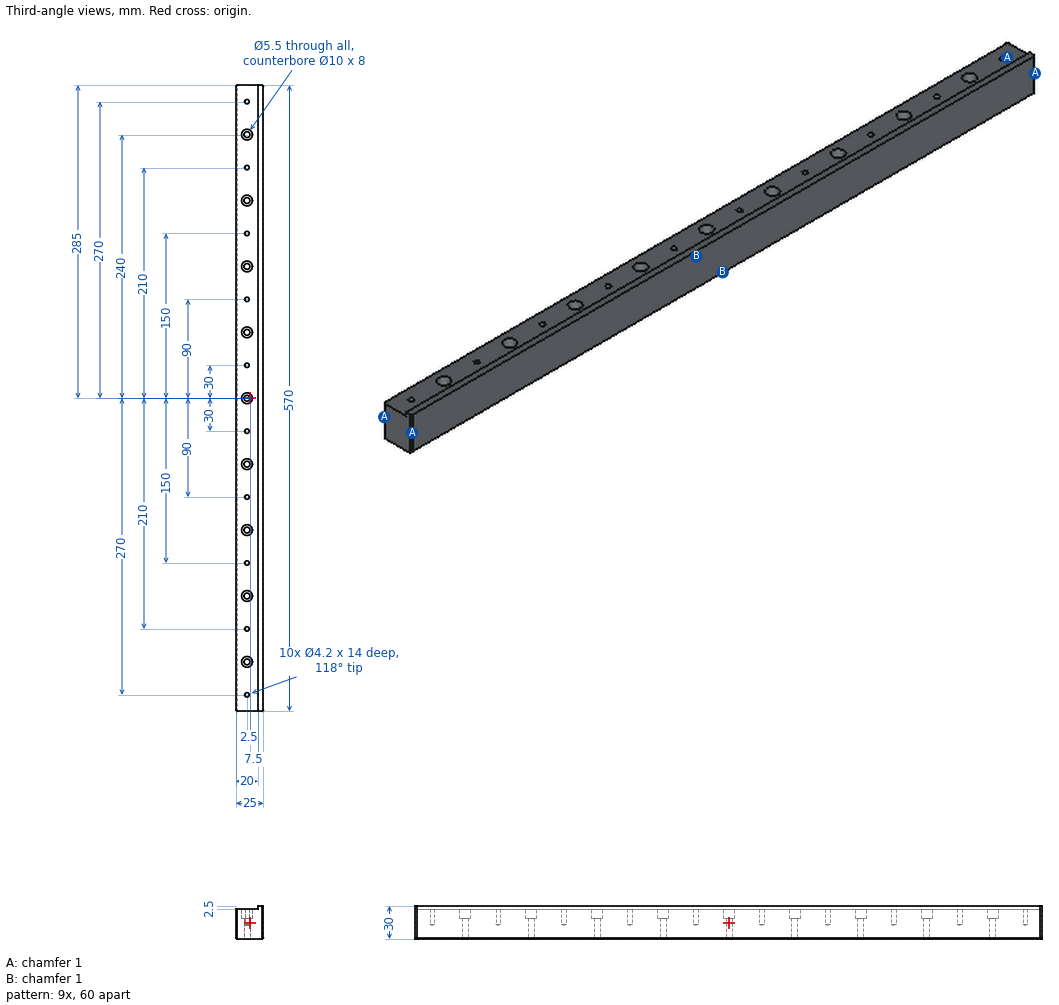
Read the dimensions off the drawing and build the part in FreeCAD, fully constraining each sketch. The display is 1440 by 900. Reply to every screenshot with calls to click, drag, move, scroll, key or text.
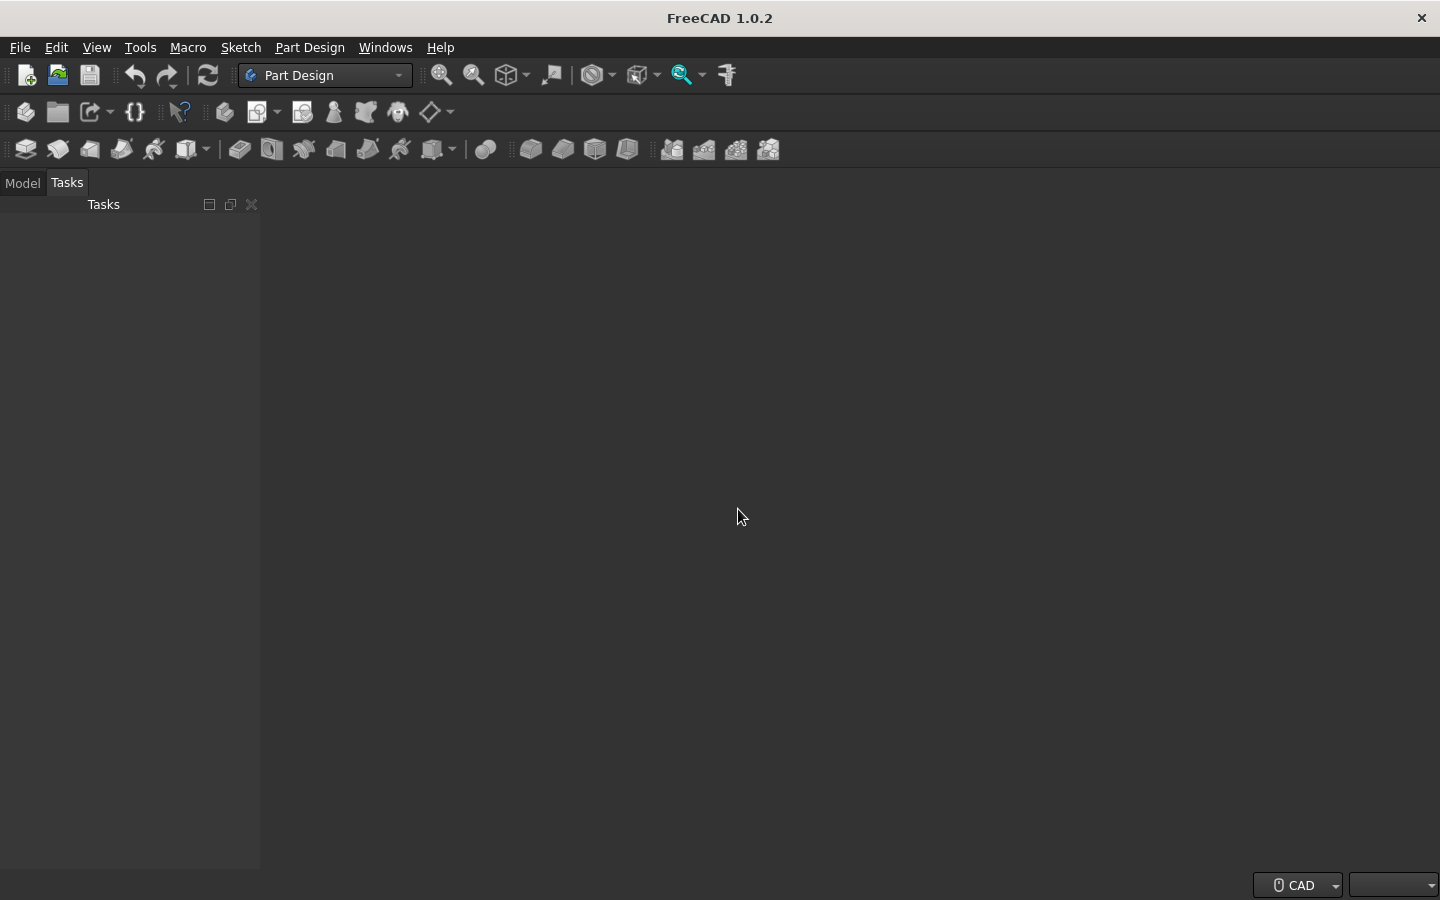
key(ctrl+n)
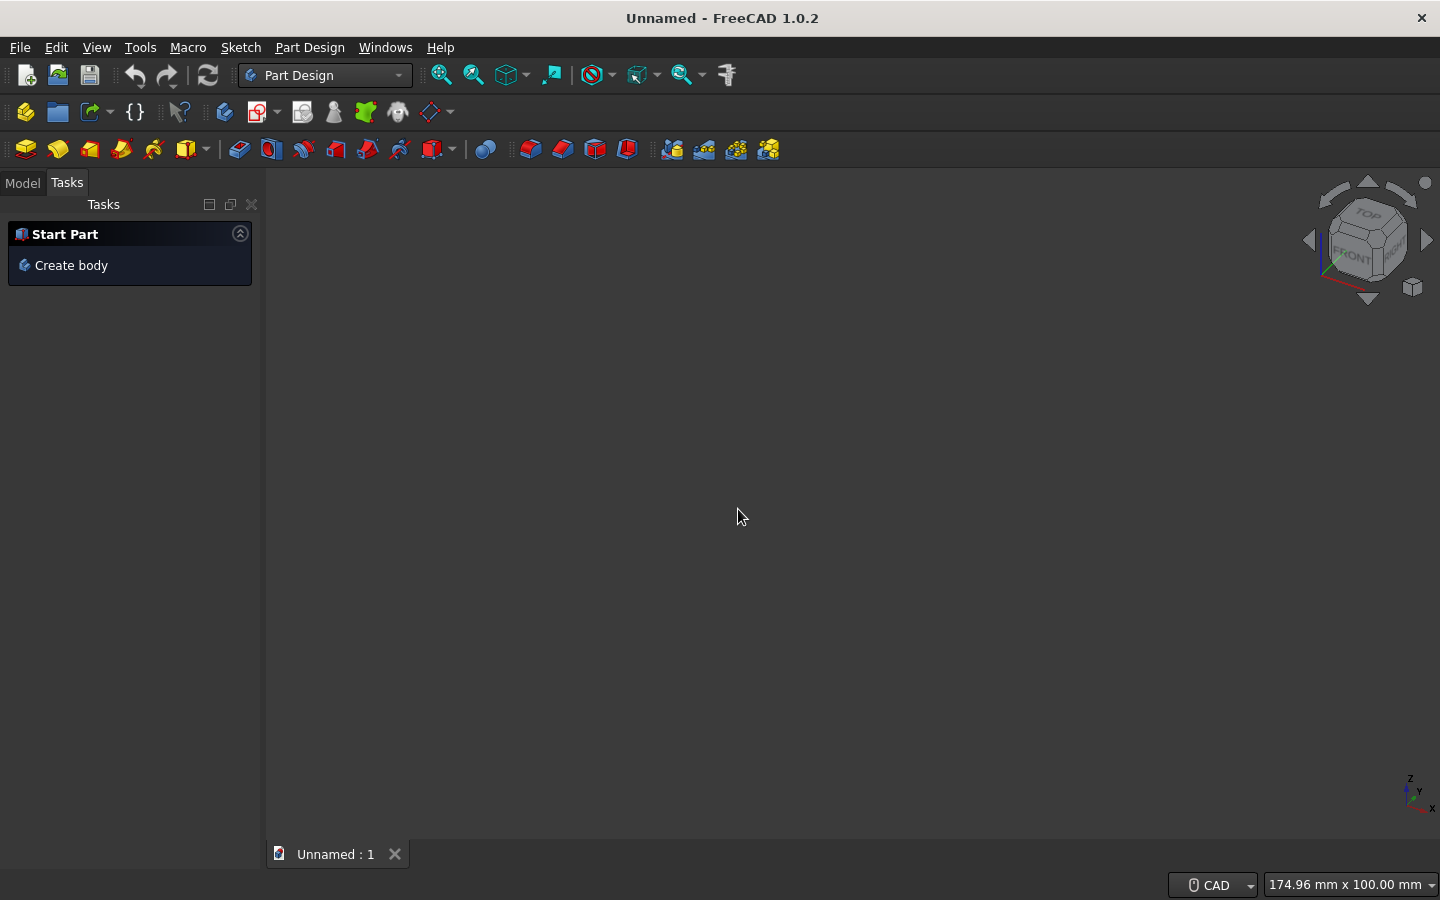
click(258, 112)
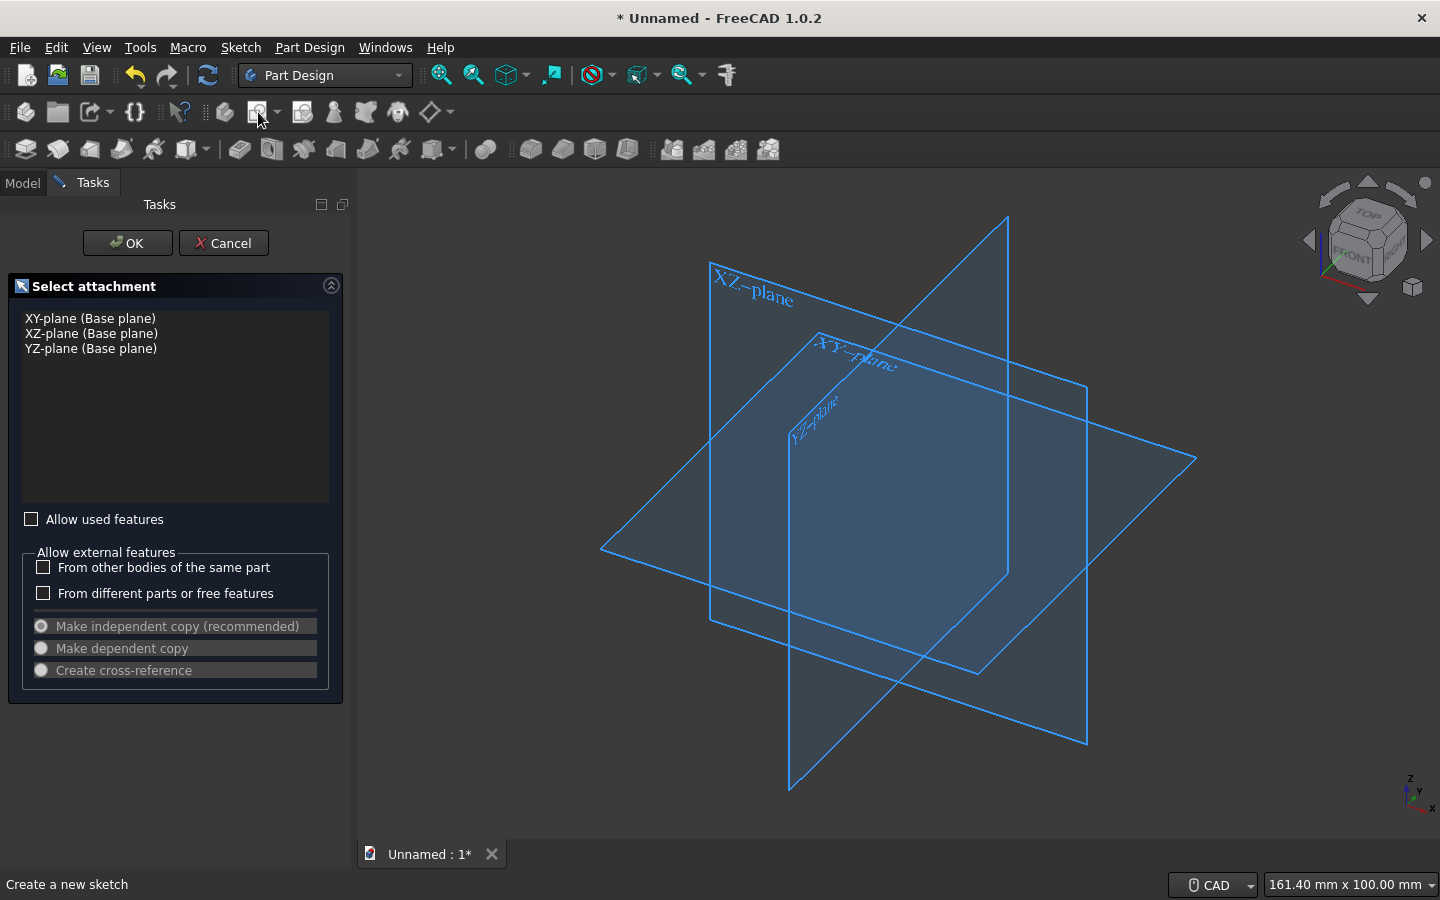
click(82, 318)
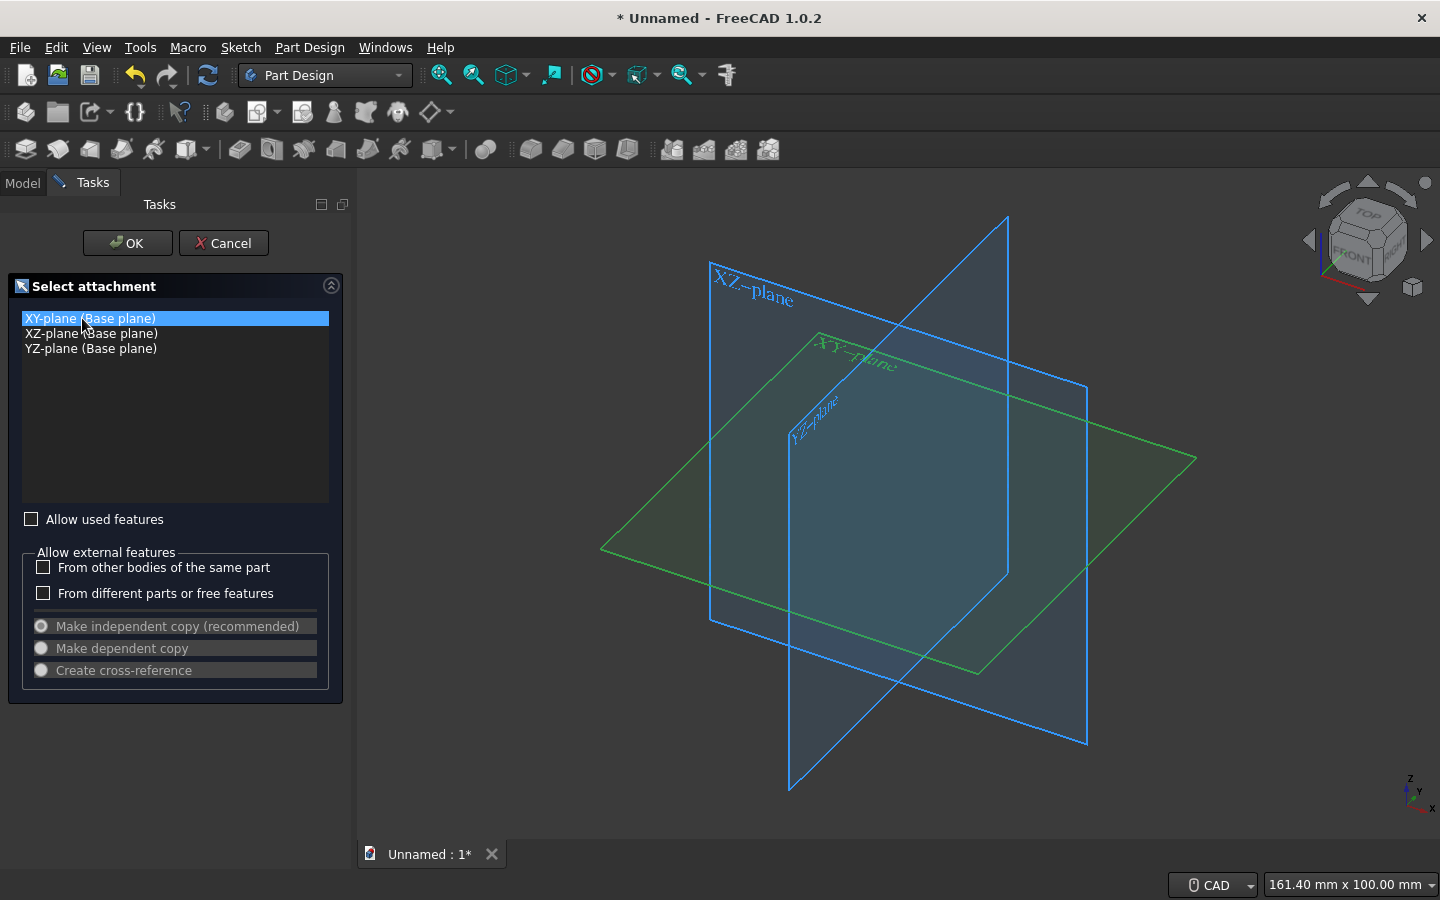
click(128, 243)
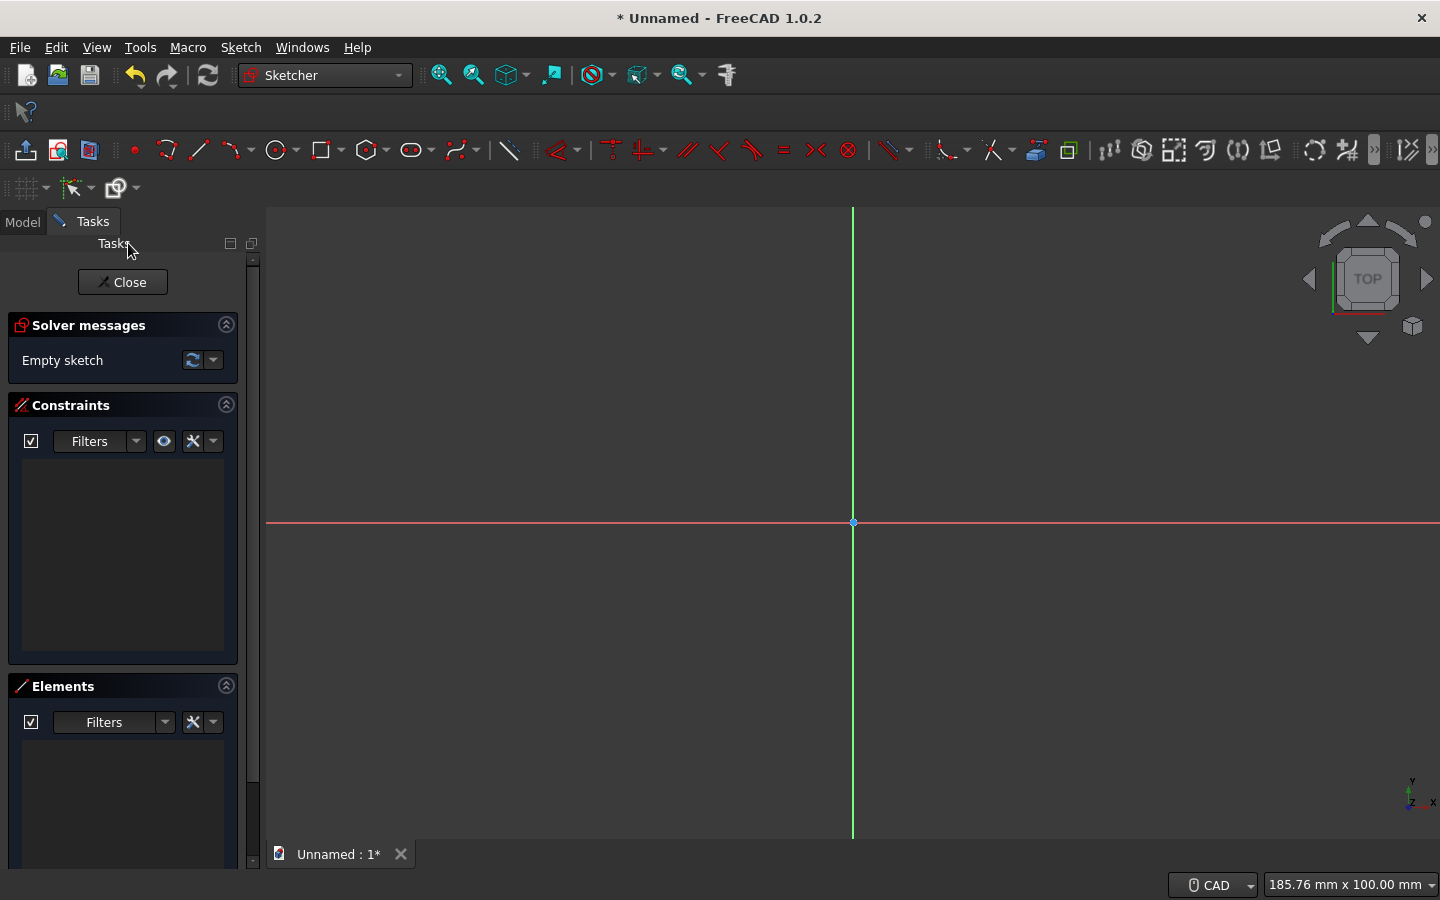
scroll(776, 523, down, 11)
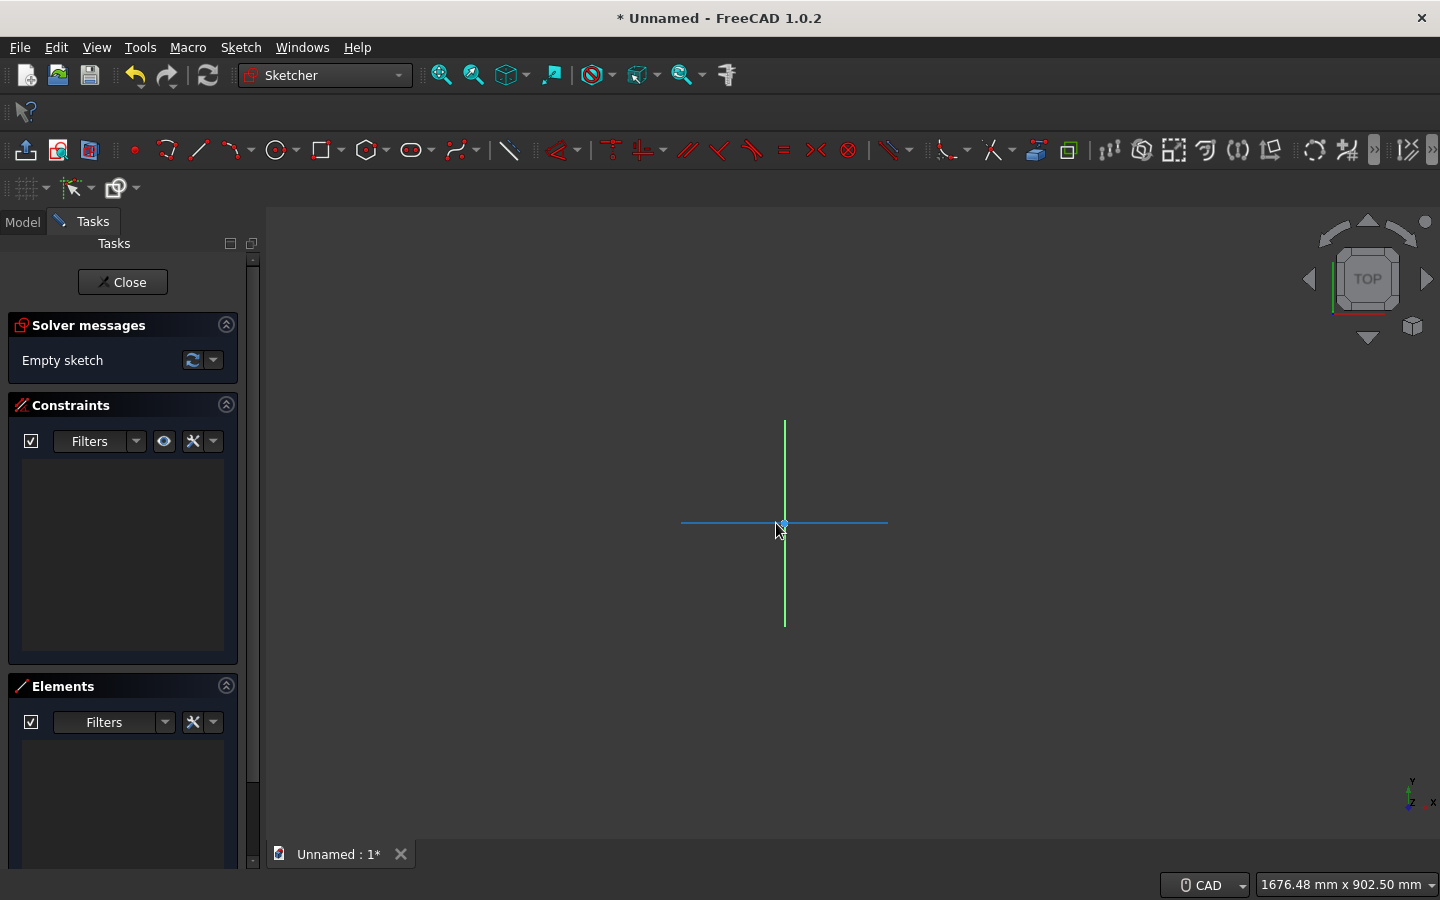
key(g)
key(v)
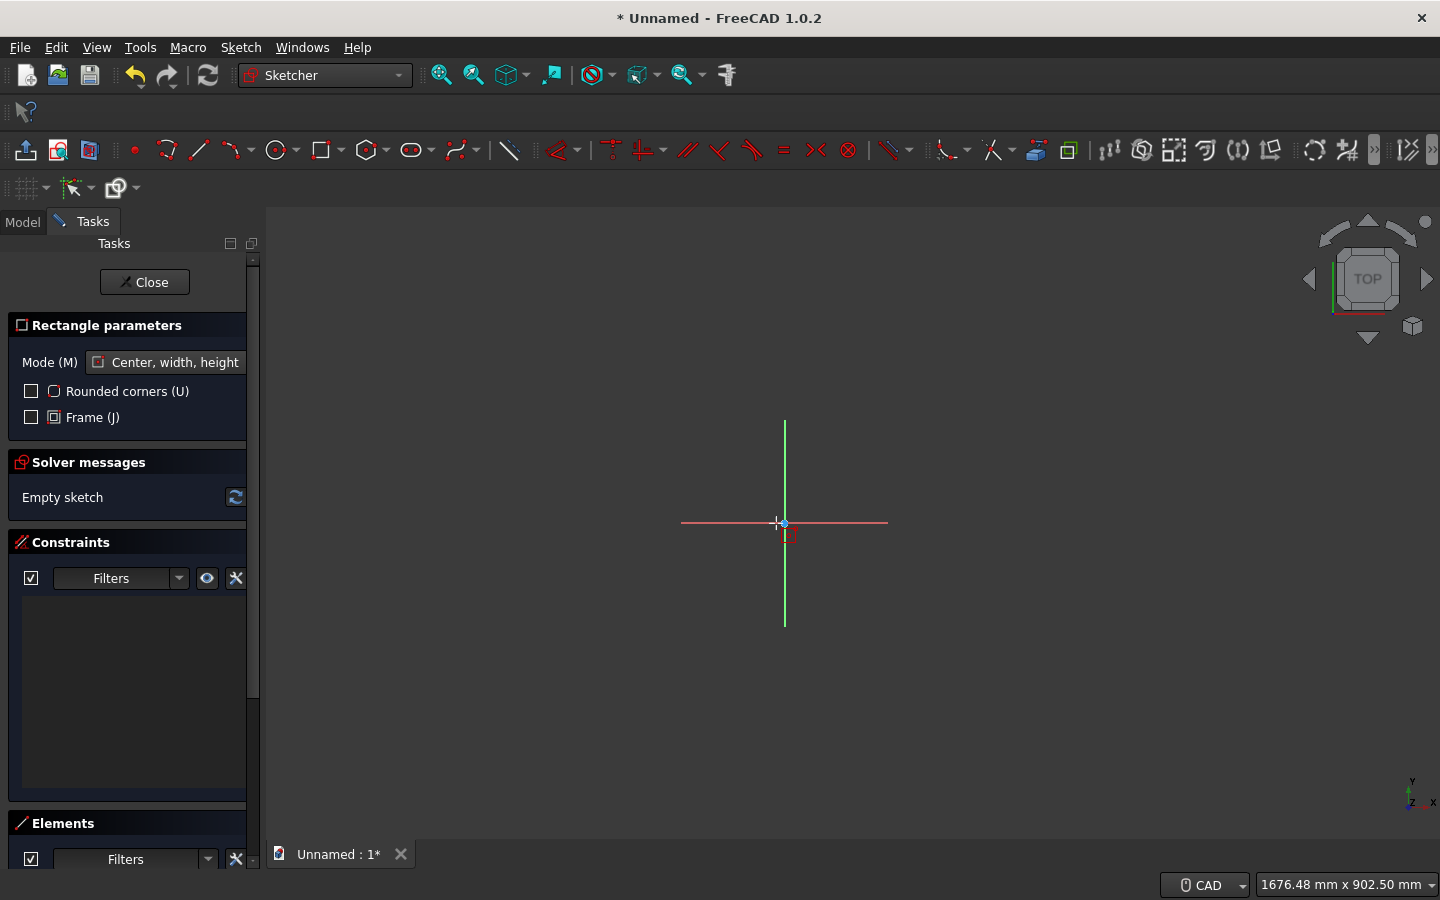
scroll(785, 523, up, 3)